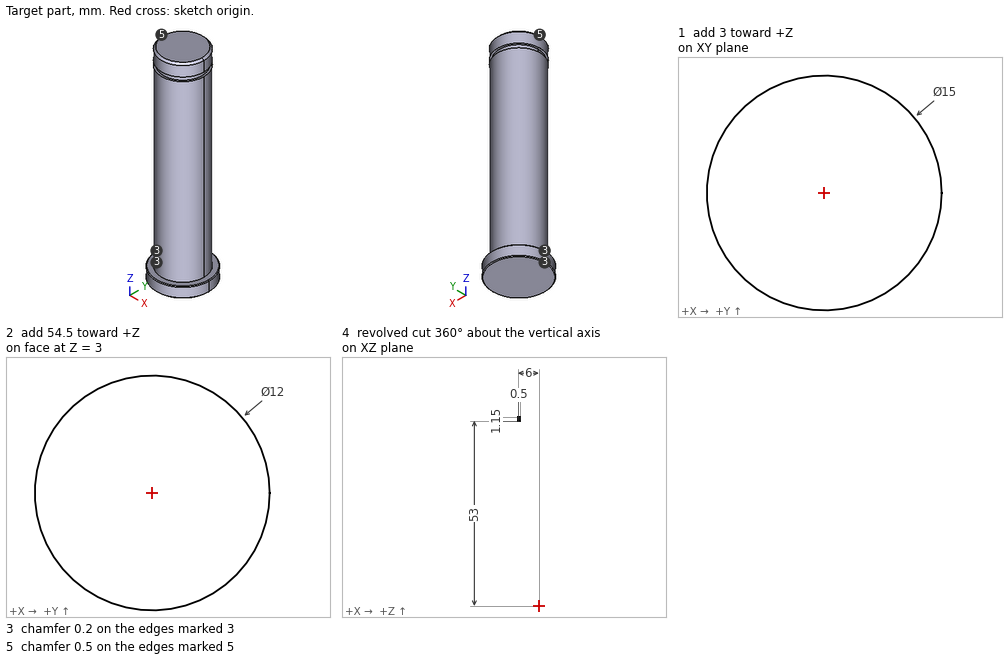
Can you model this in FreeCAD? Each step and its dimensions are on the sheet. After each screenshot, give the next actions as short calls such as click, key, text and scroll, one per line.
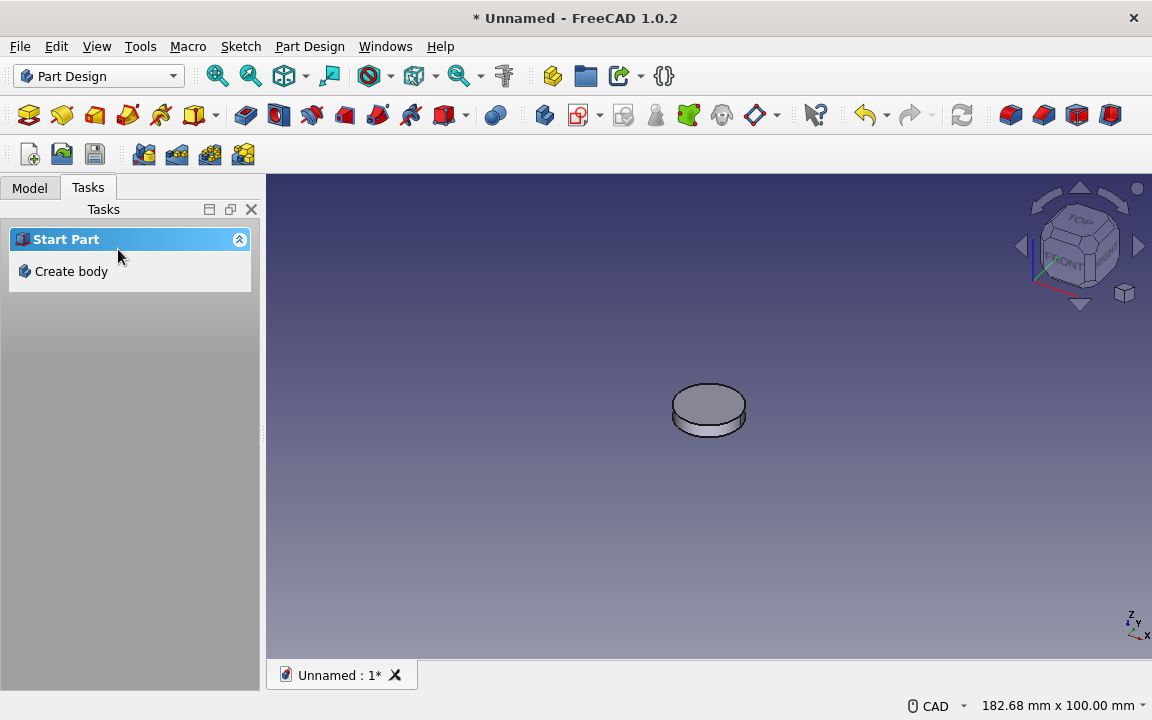
click(218, 76)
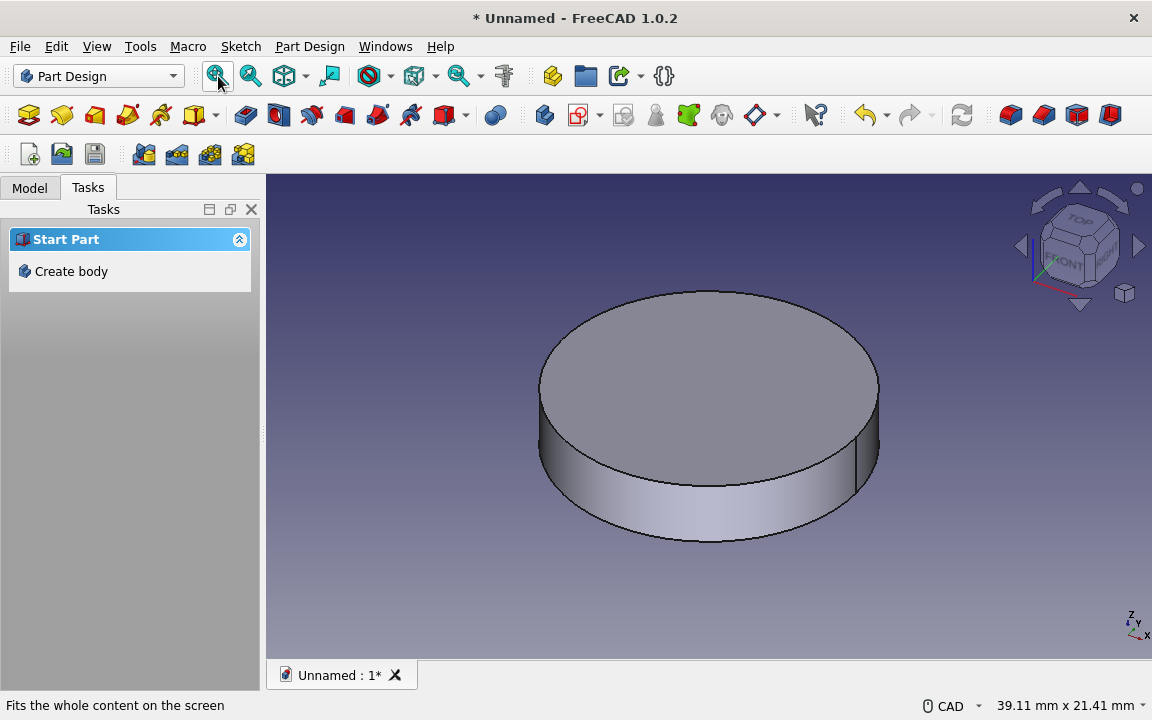
click(709, 388)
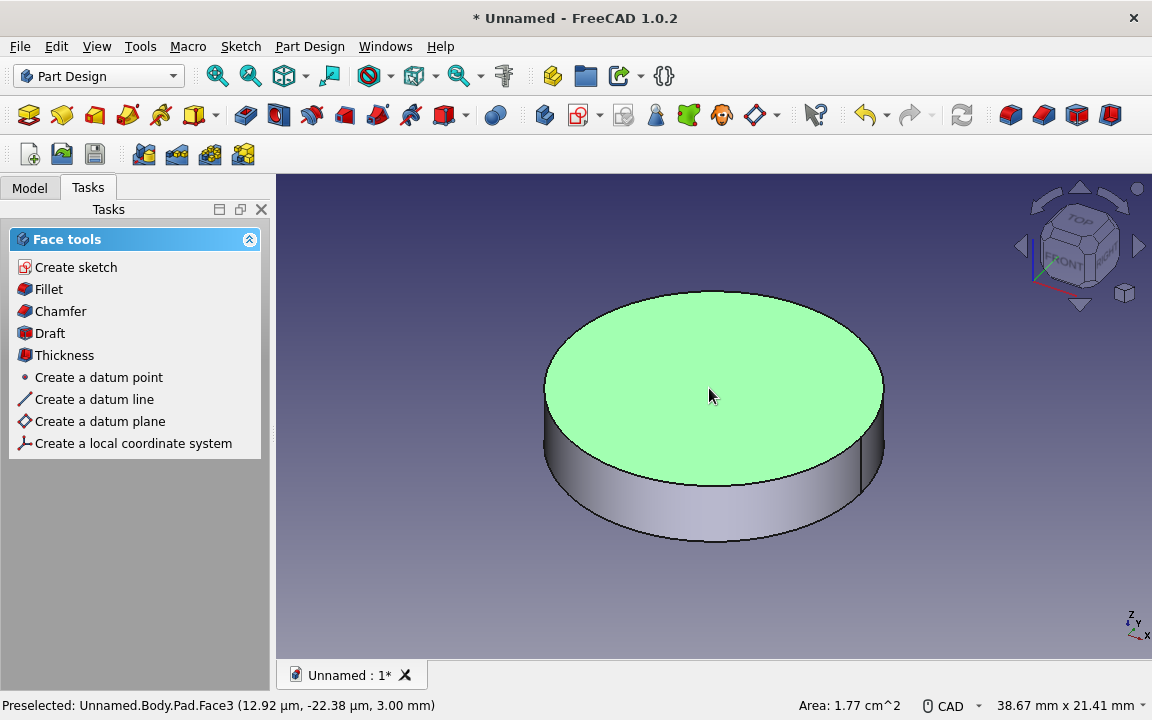
click(578, 116)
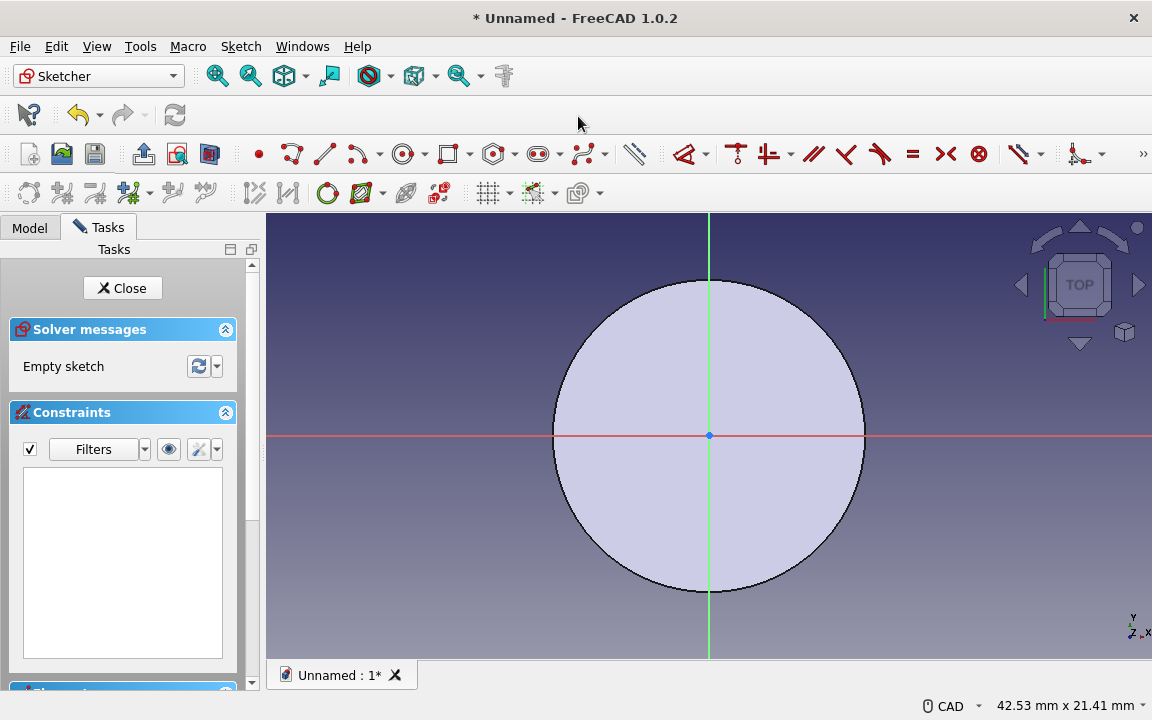
key(g)
key(c)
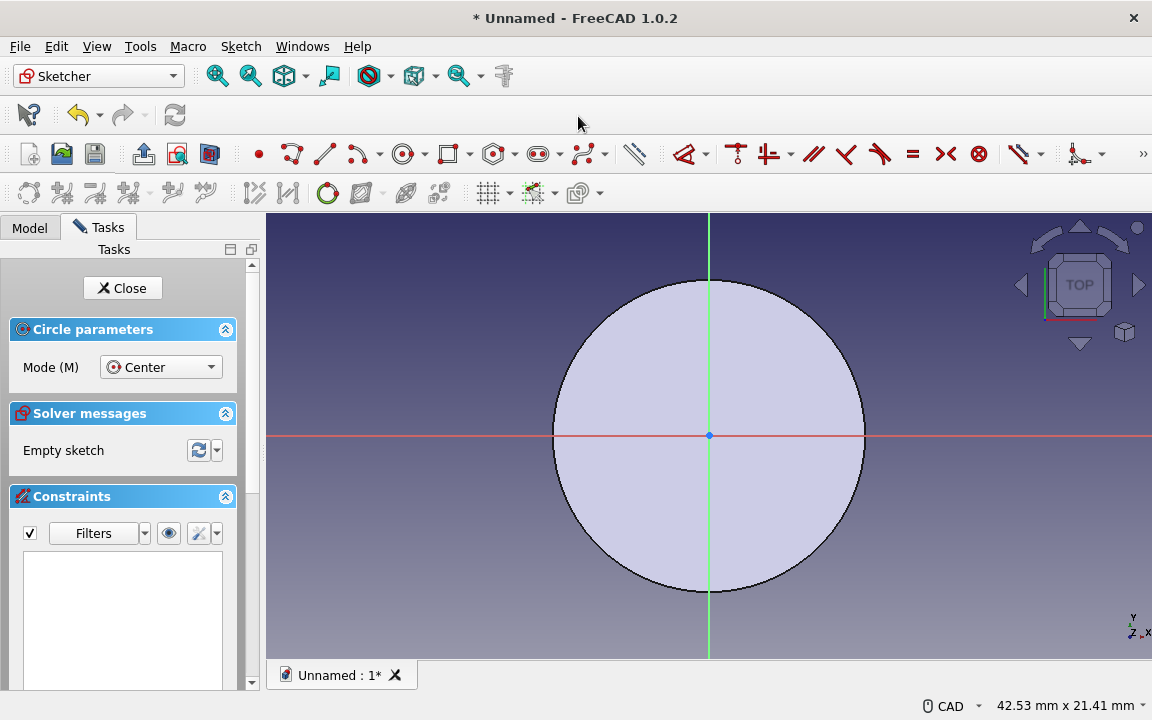
click(709, 436)
move(797, 348)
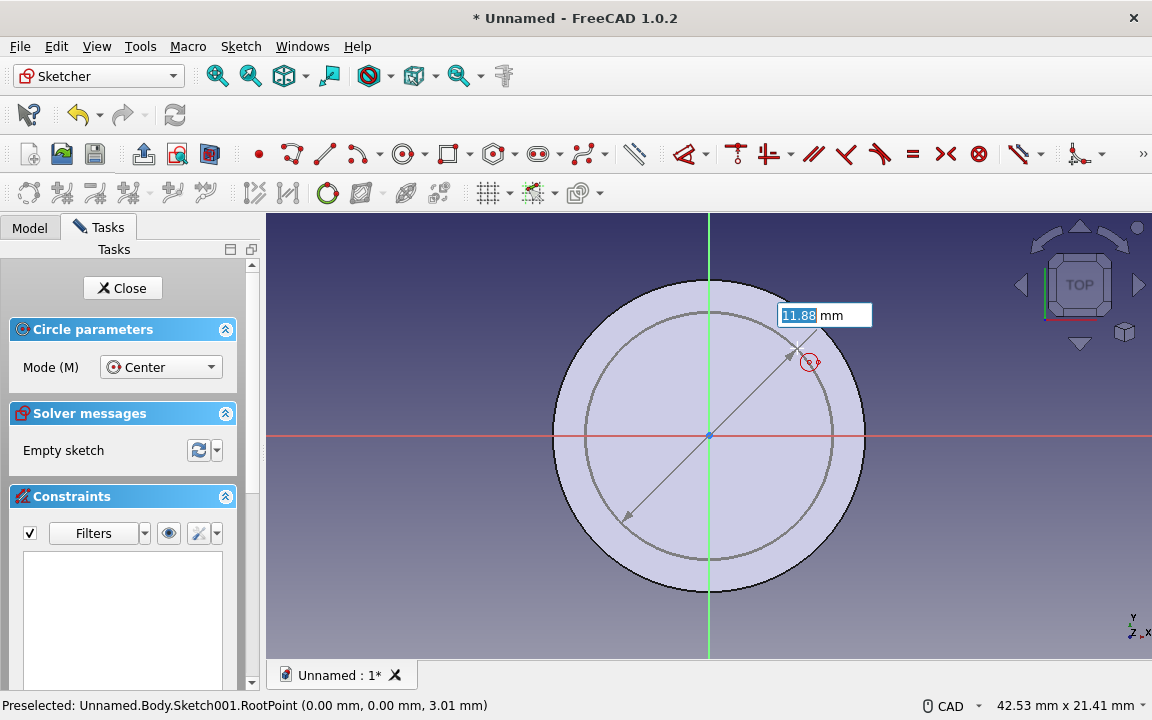
text(12)
key(Return)
key(Escape)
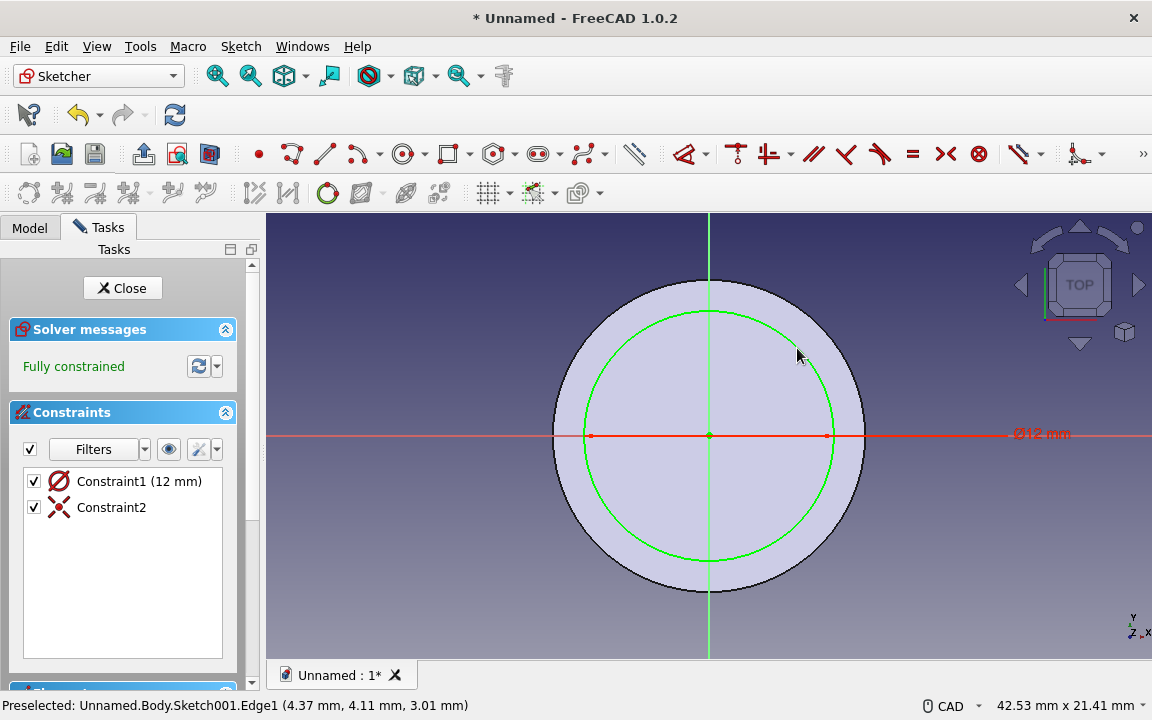
click(123, 288)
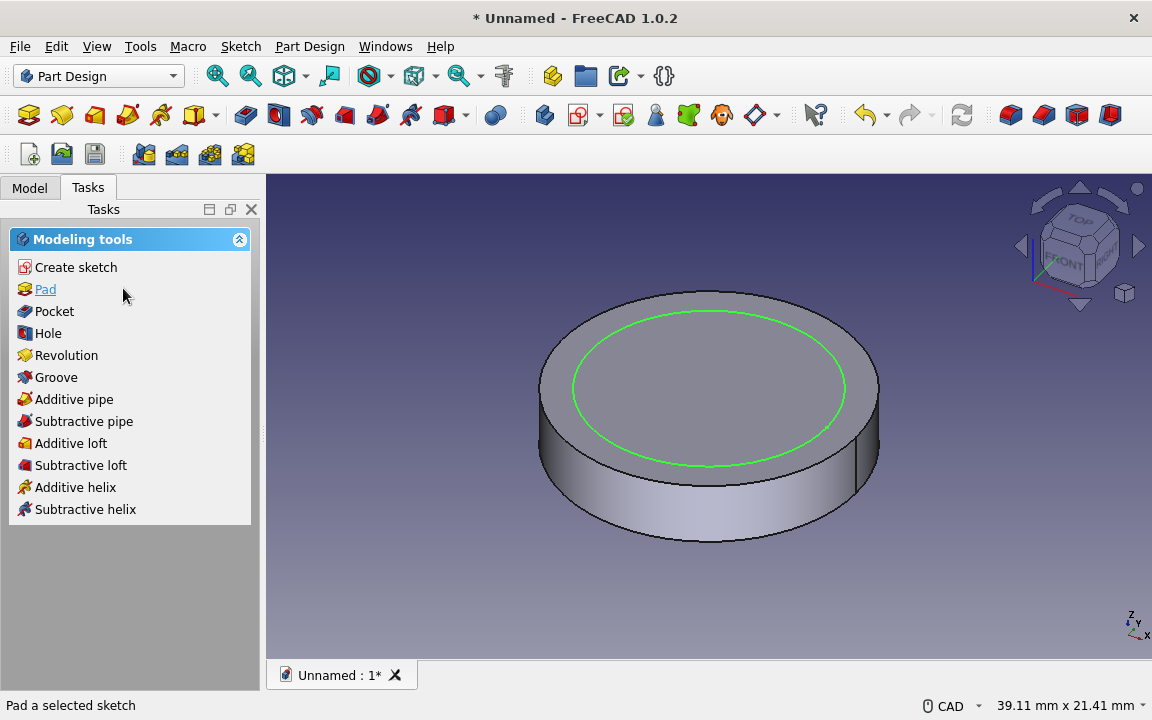
click(29, 116)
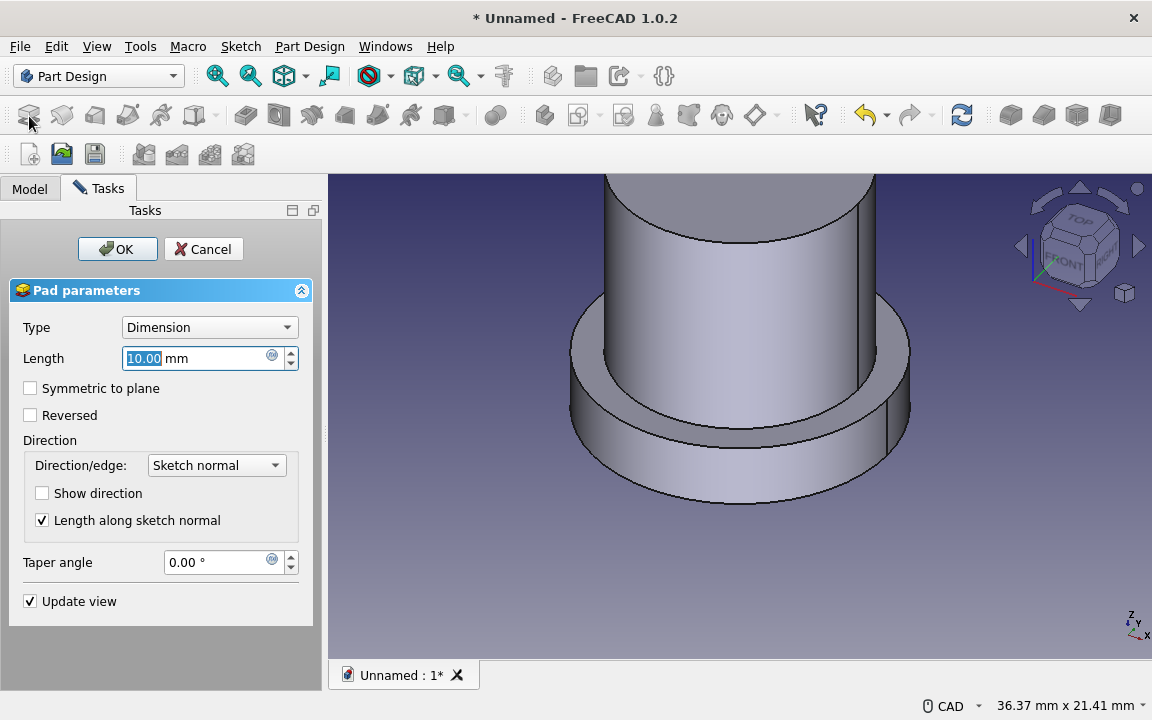
text(54.5)
key(Tab)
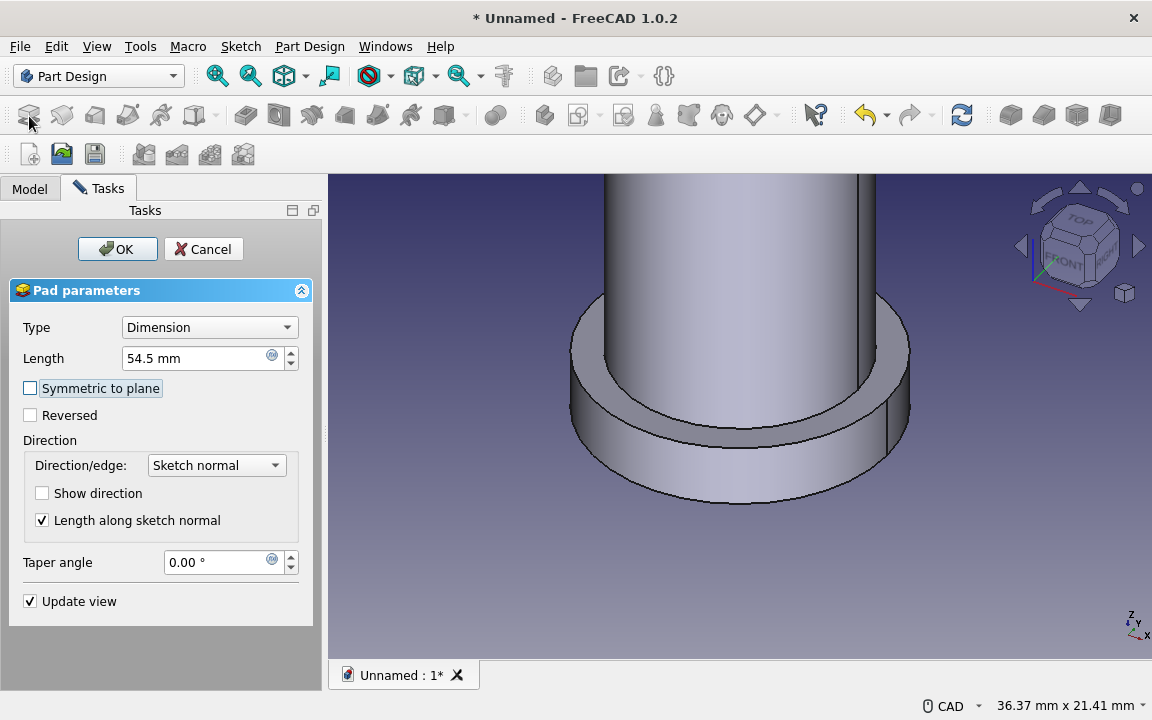
click(118, 249)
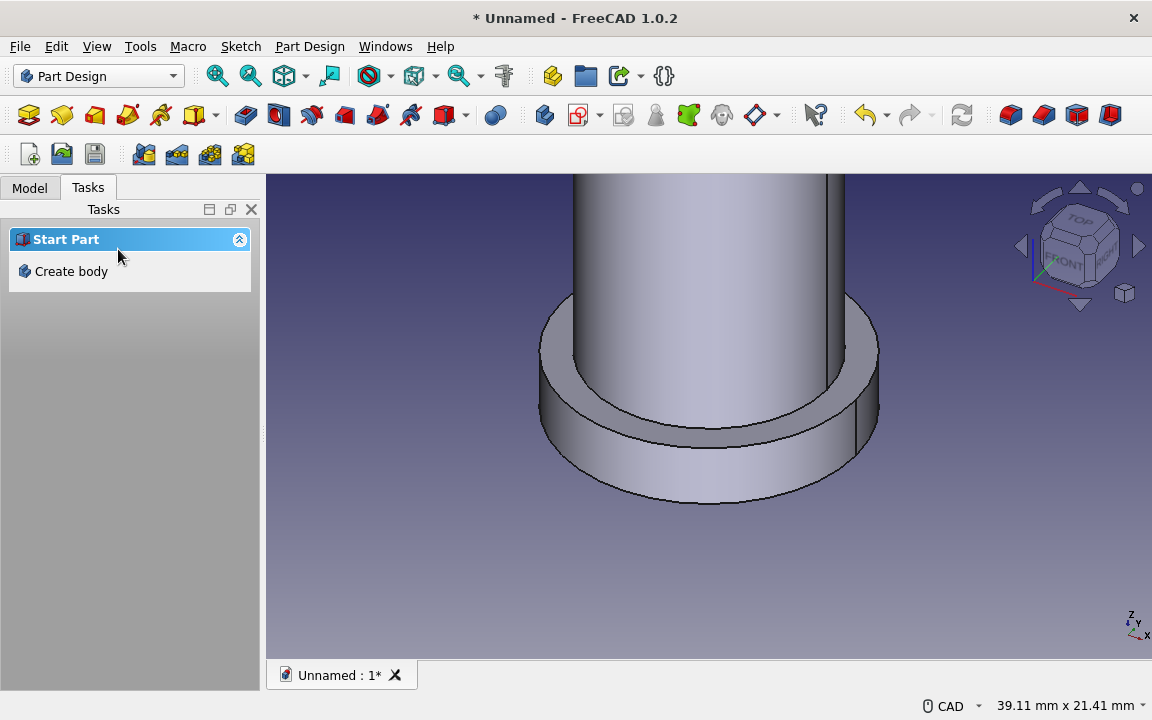
key(v)
key(f)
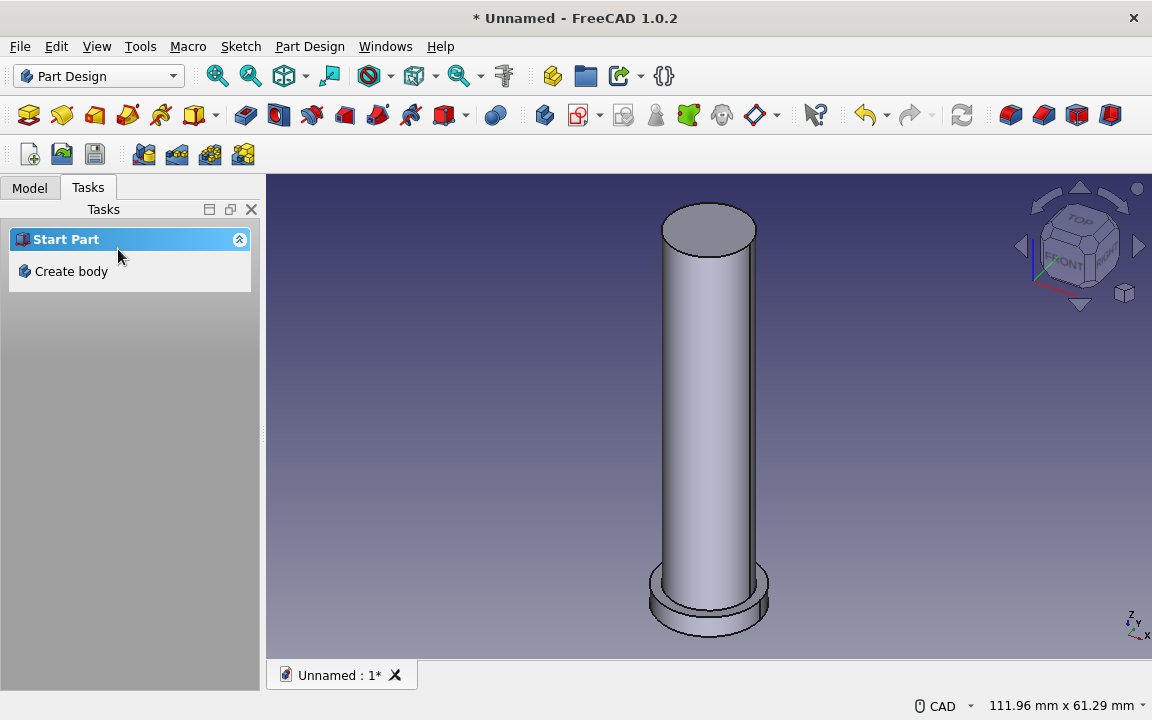
click(650, 586)